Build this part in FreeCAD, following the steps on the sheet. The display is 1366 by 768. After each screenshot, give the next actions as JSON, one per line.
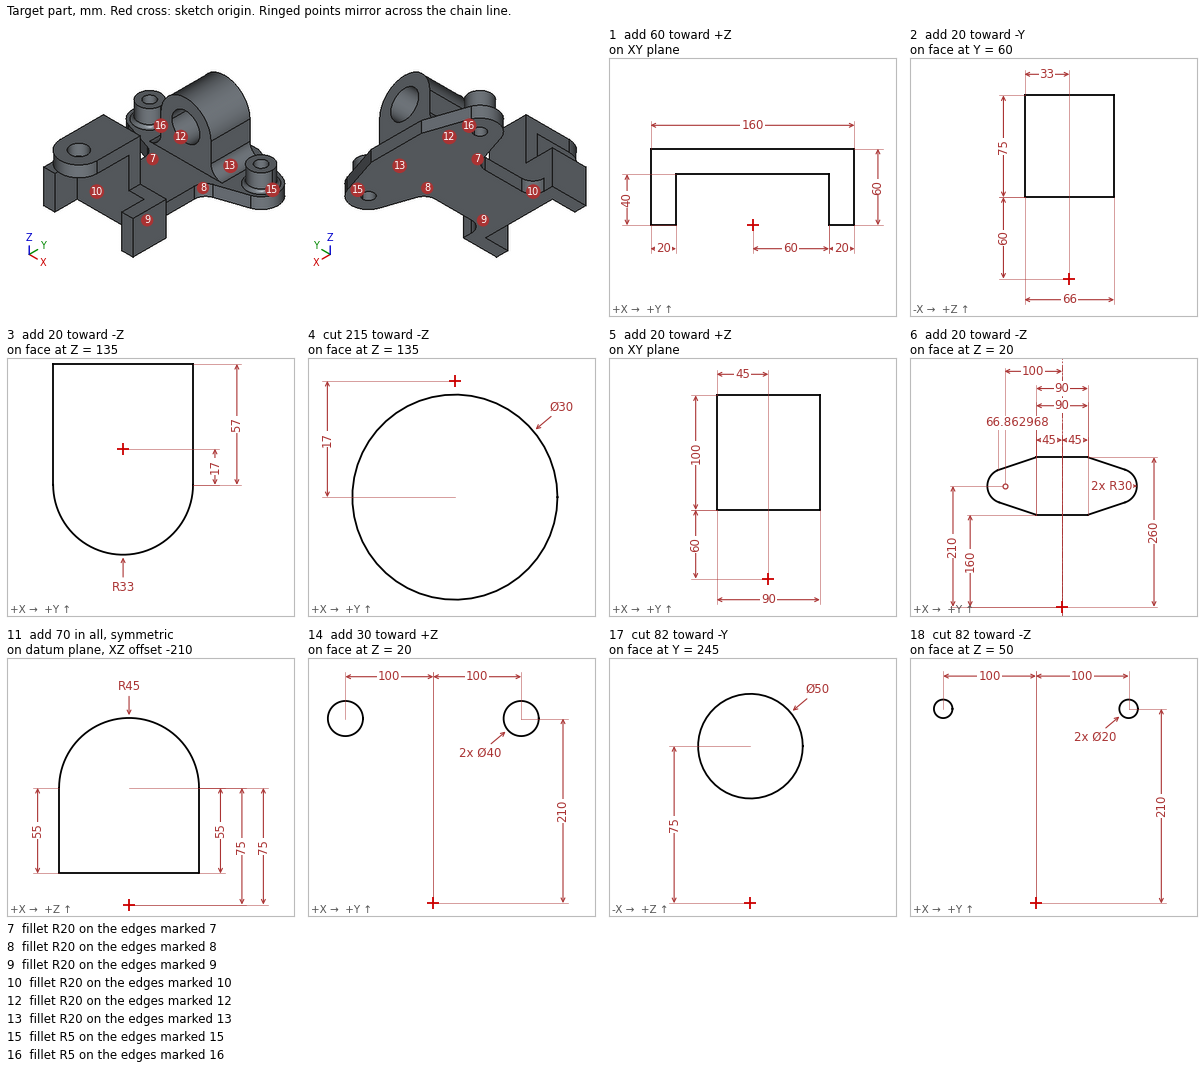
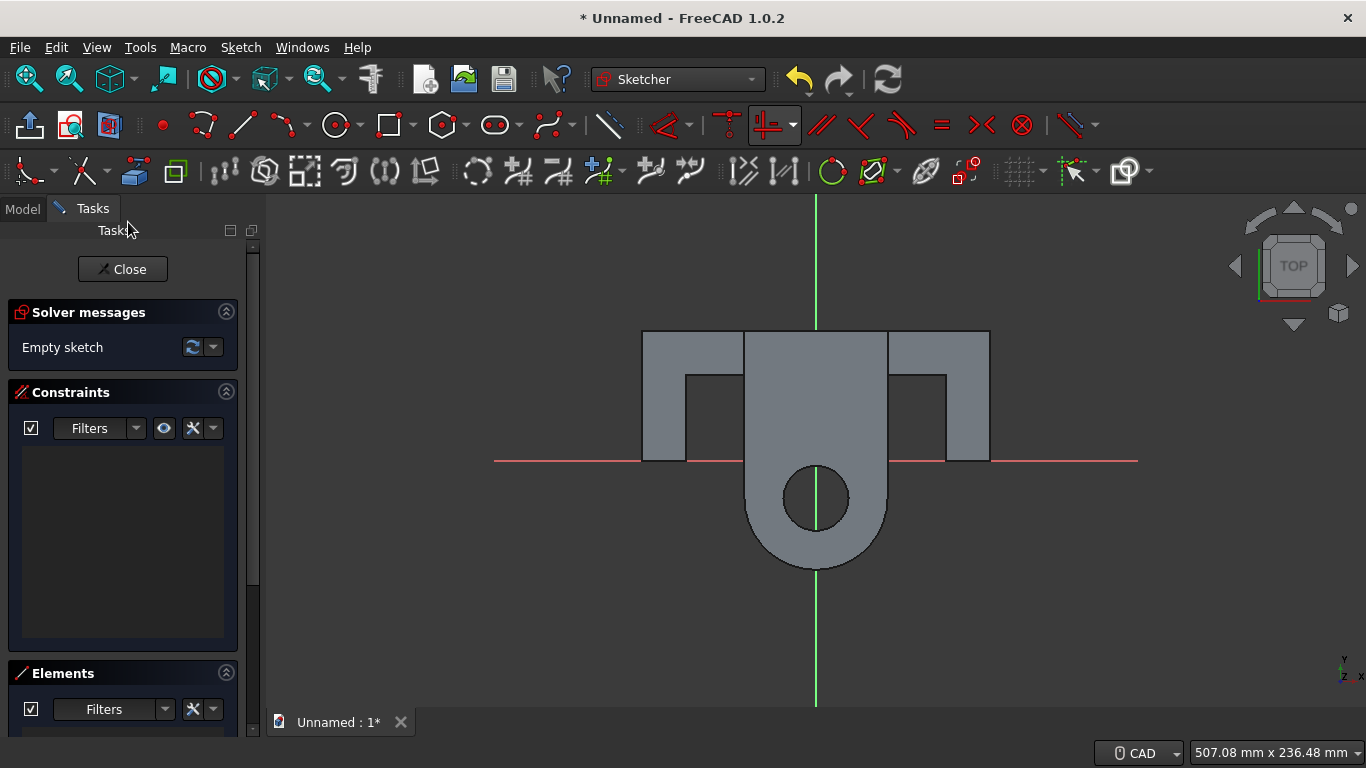
{"action": "key", "text": "q s"}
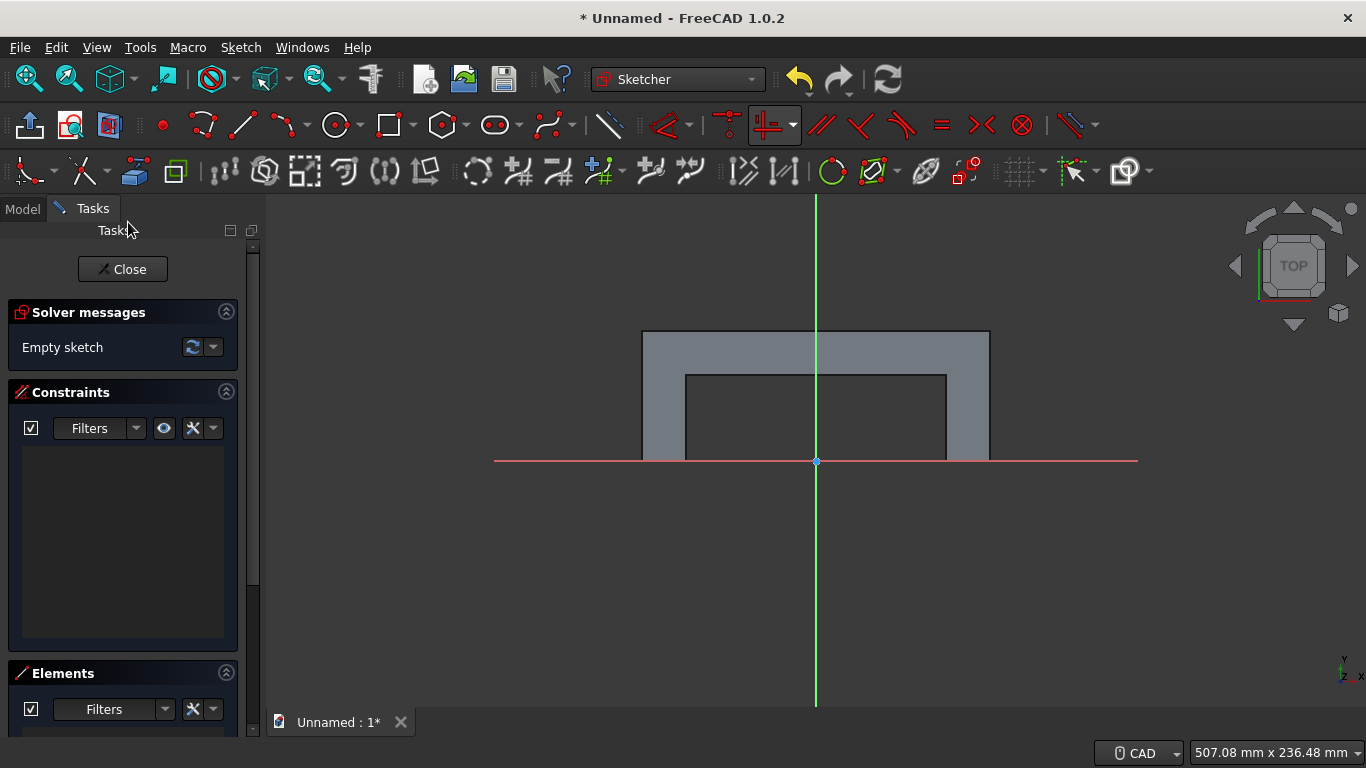
{"action": "scroll", "coordinate": [608, 679], "scroll_direction": "down", "scroll_amount": 2}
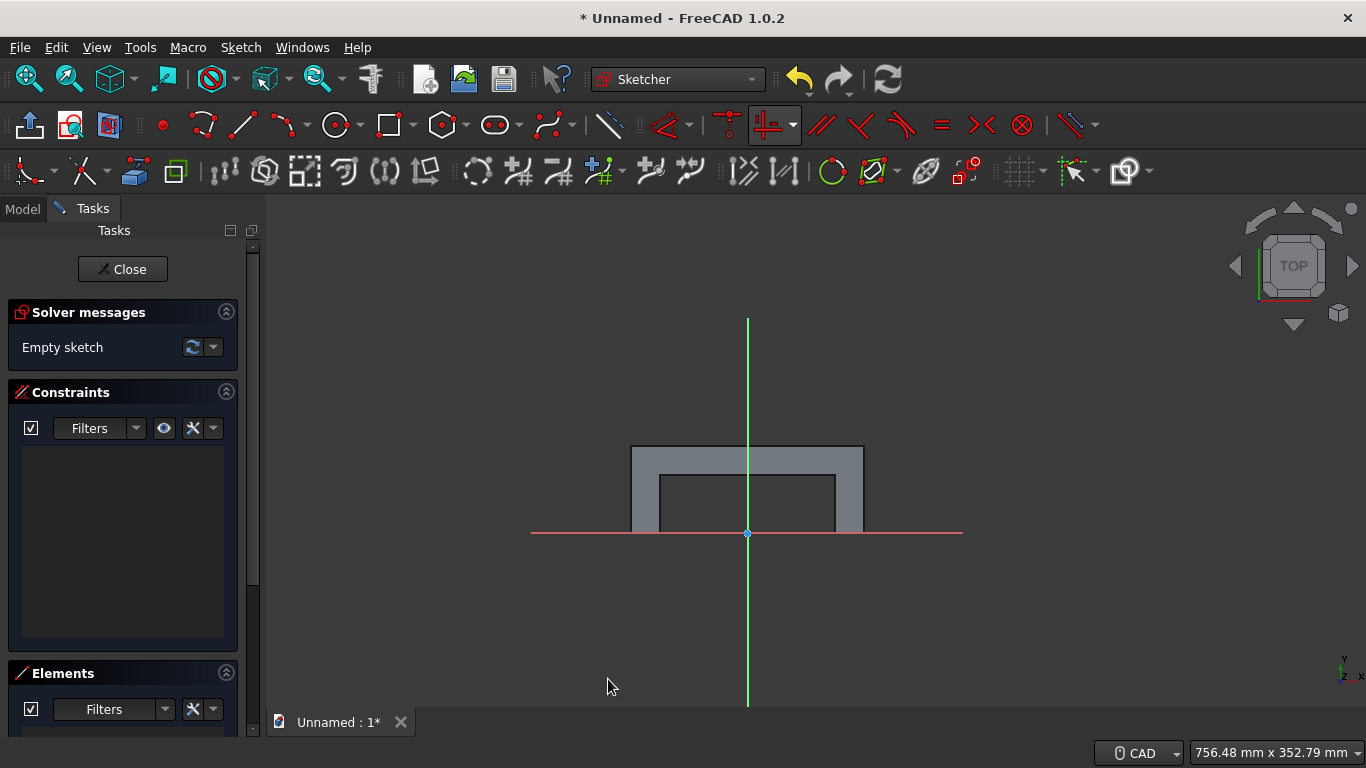
{"action": "scroll", "coordinate": [748, 349], "scroll_direction": "up", "scroll_amount": 2}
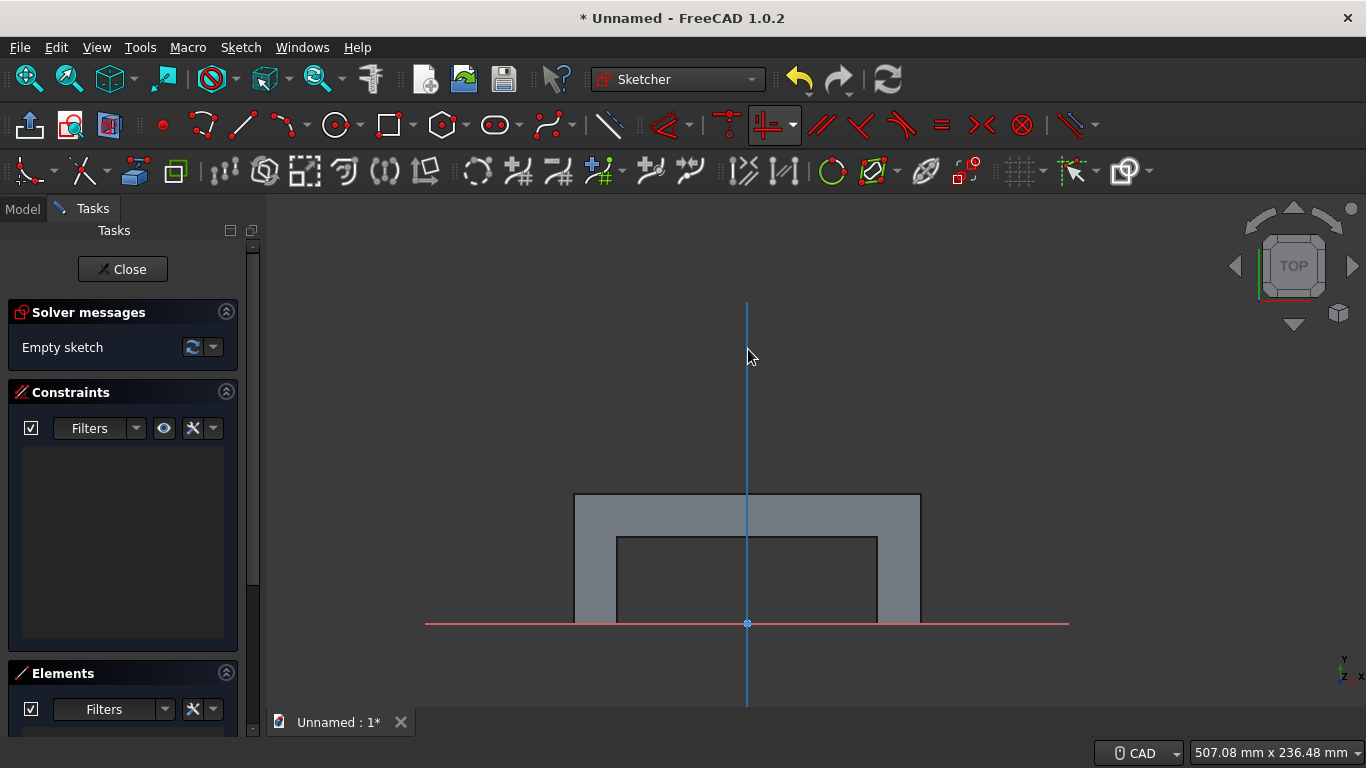
{"action": "key", "text": "g r"}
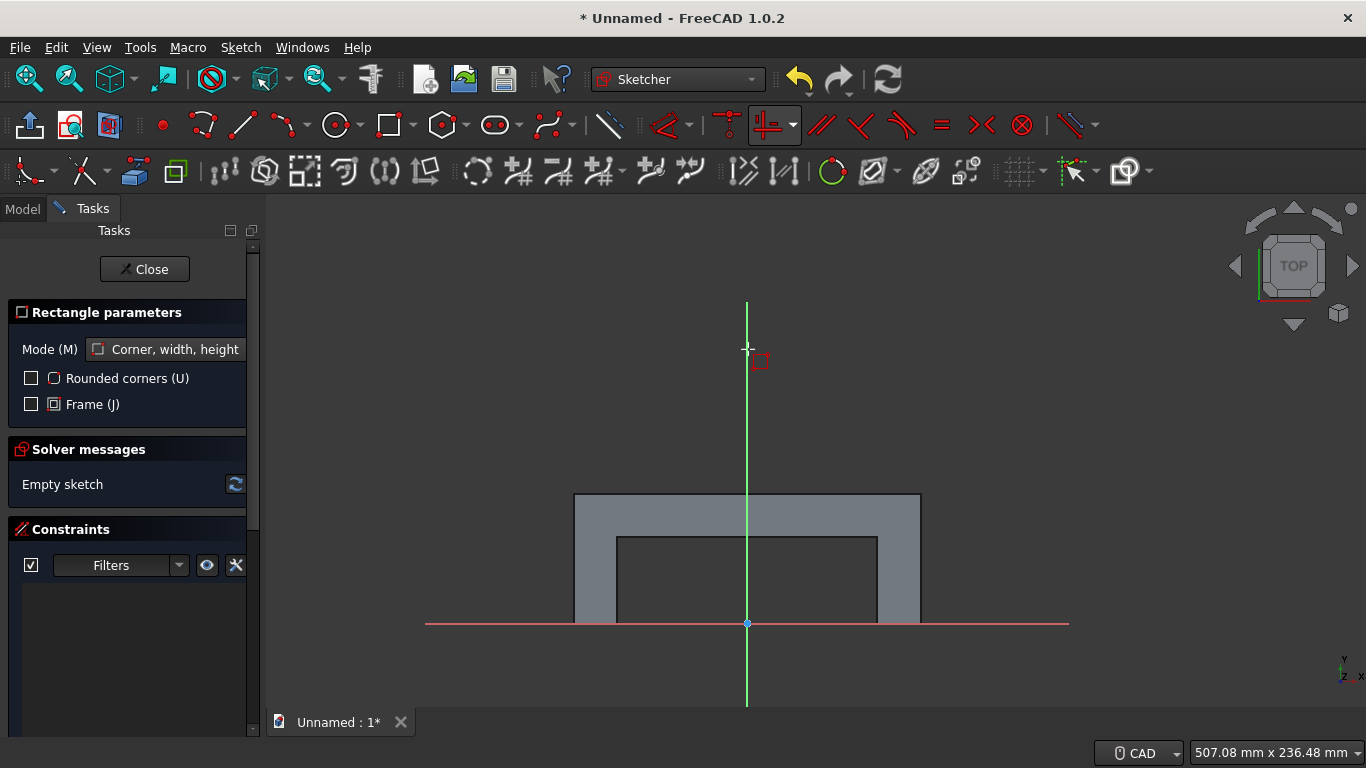
{"action": "left_click", "coordinate": [649, 277]}
{"action": "left_click", "coordinate": [845, 494]}
{"action": "key", "text": "Escape"}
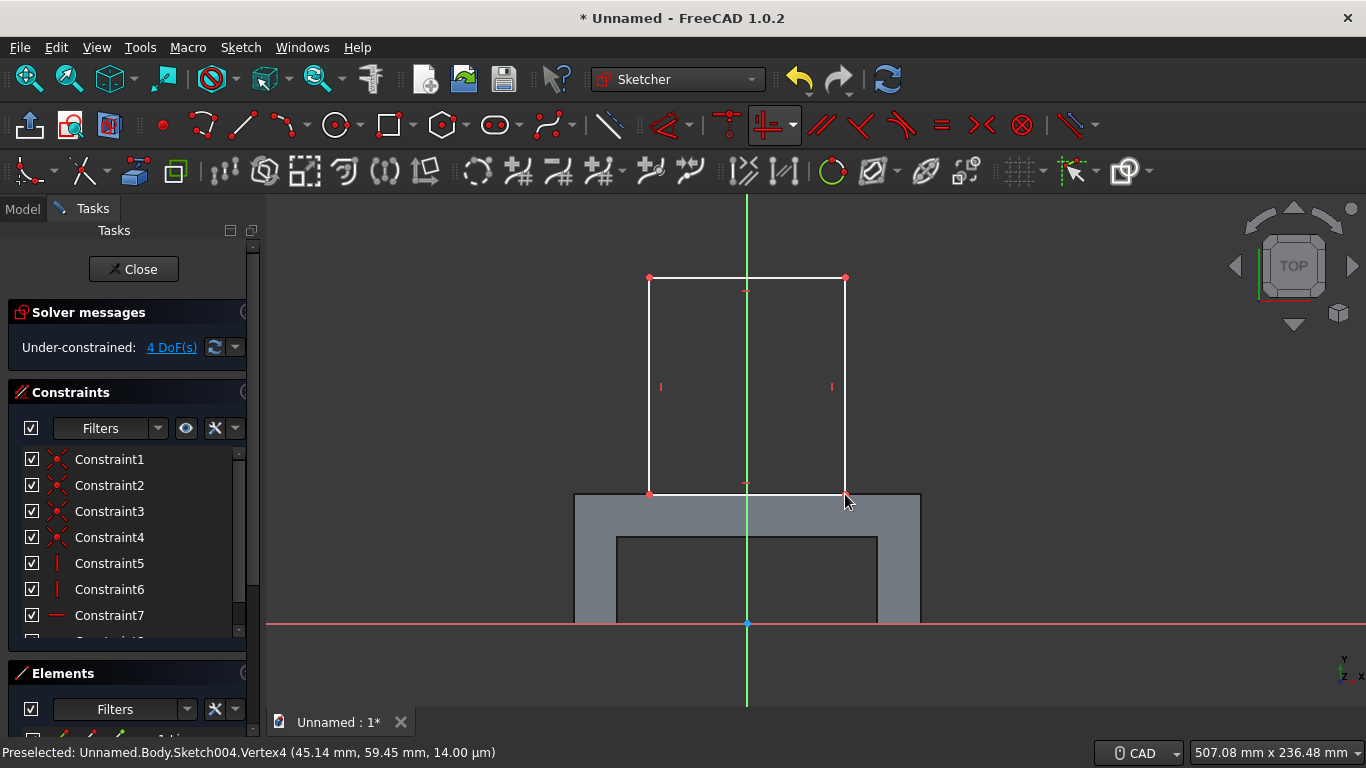
{"action": "key", "text": "d"}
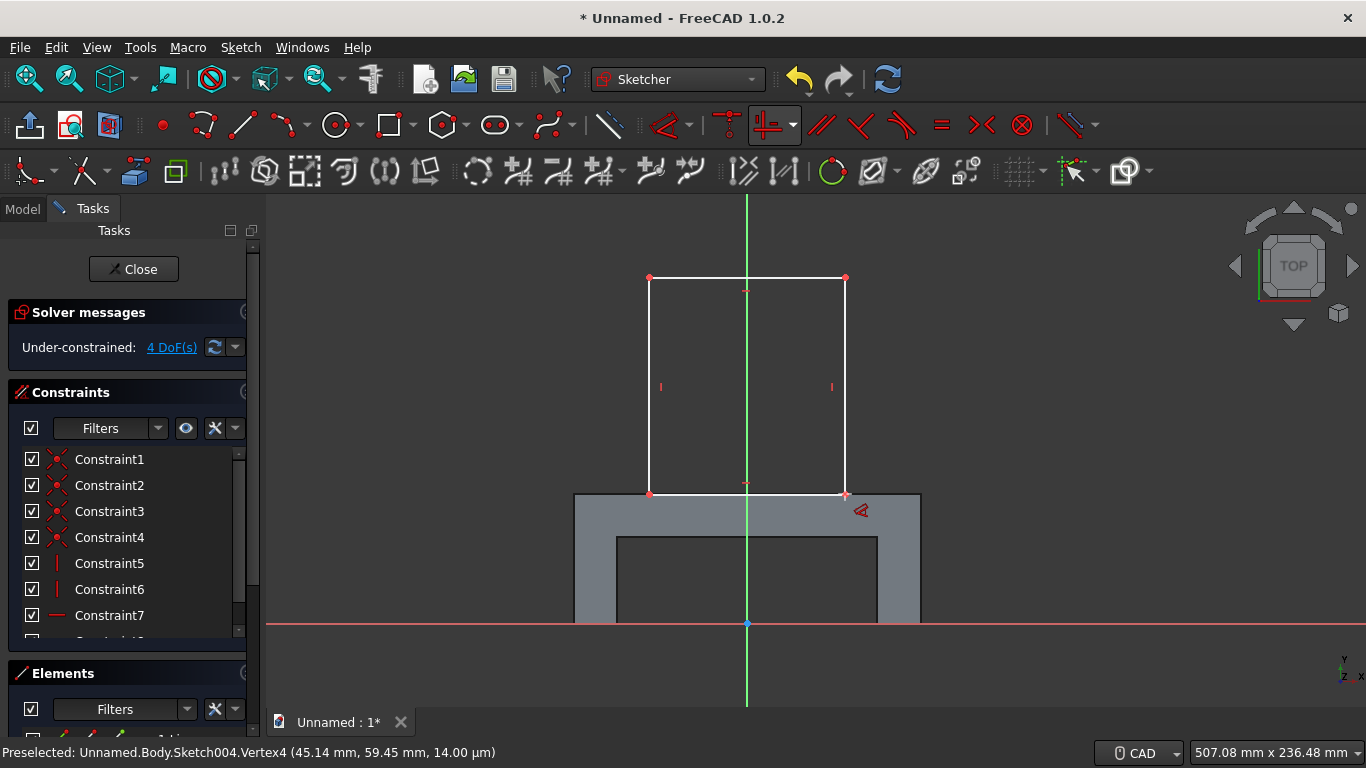
{"action": "left_click", "coordinate": [708, 495]}
{"action": "left_click", "coordinate": [702, 529]}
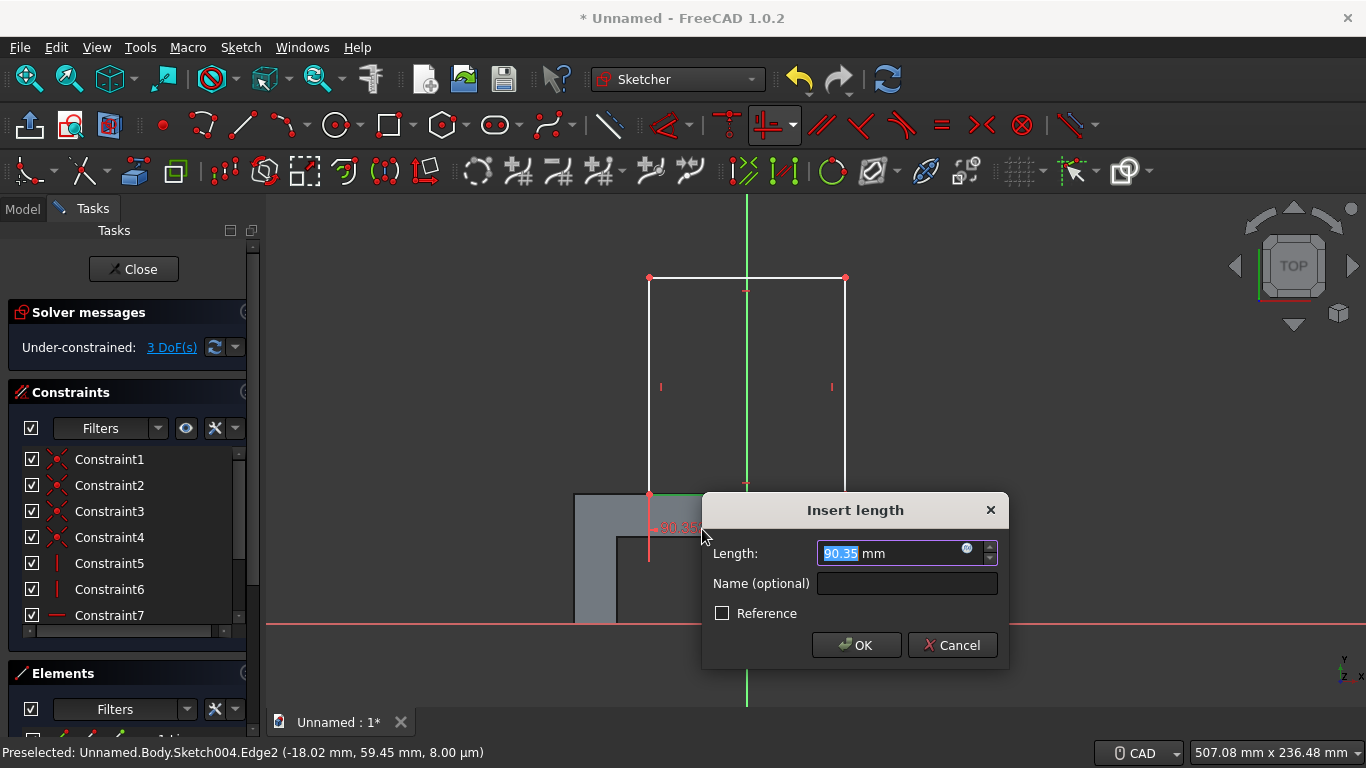
{"action": "type", "text": "90"}
{"action": "key", "text": "Return"}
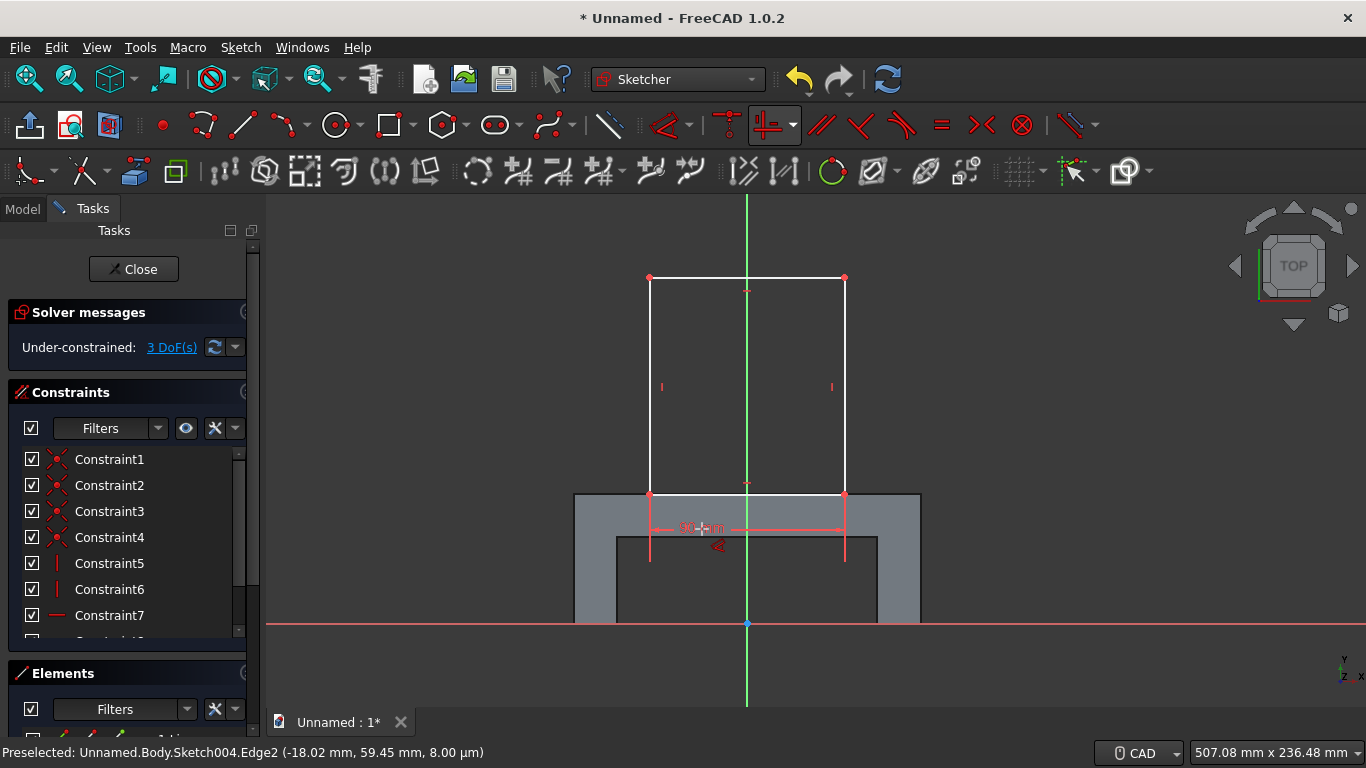
{"action": "left_click", "coordinate": [650, 343]}
{"action": "left_click", "coordinate": [616, 386]}